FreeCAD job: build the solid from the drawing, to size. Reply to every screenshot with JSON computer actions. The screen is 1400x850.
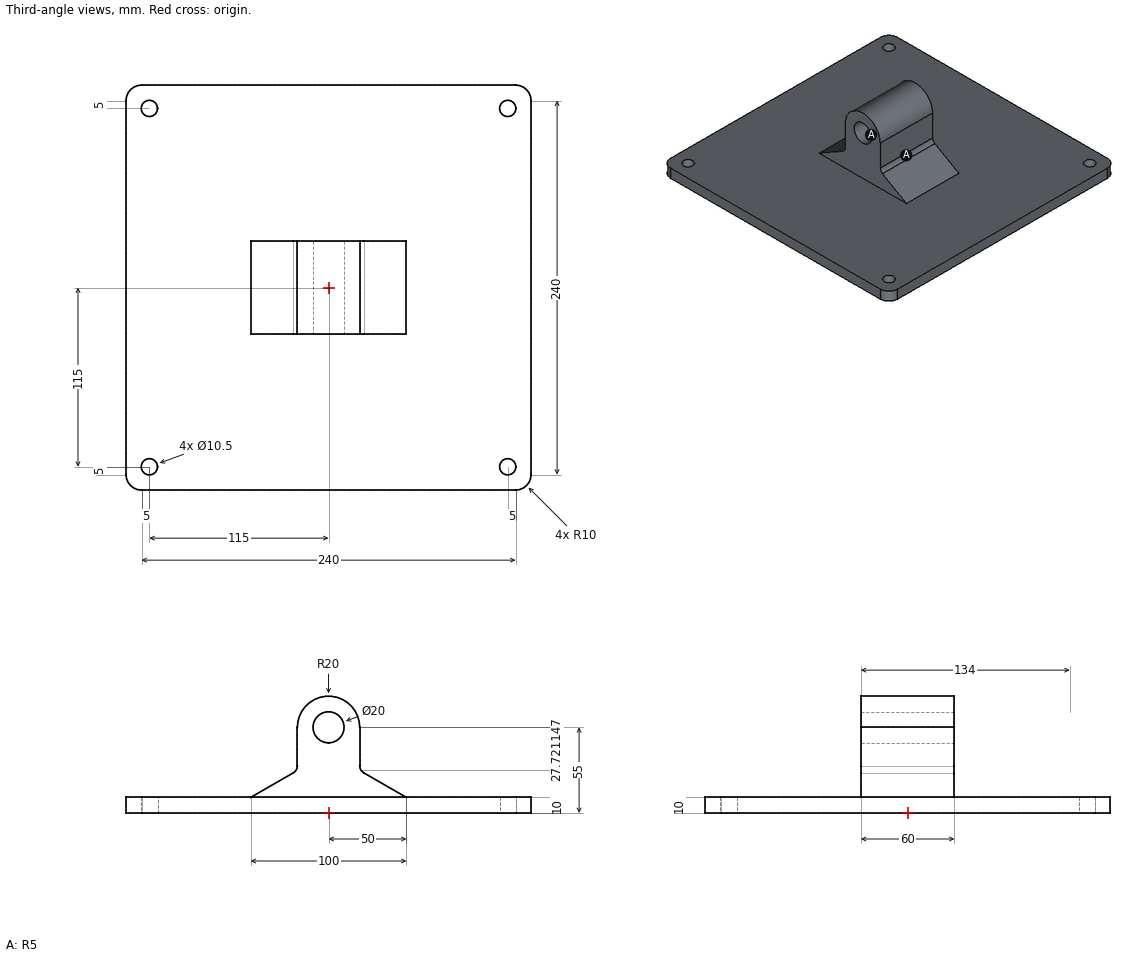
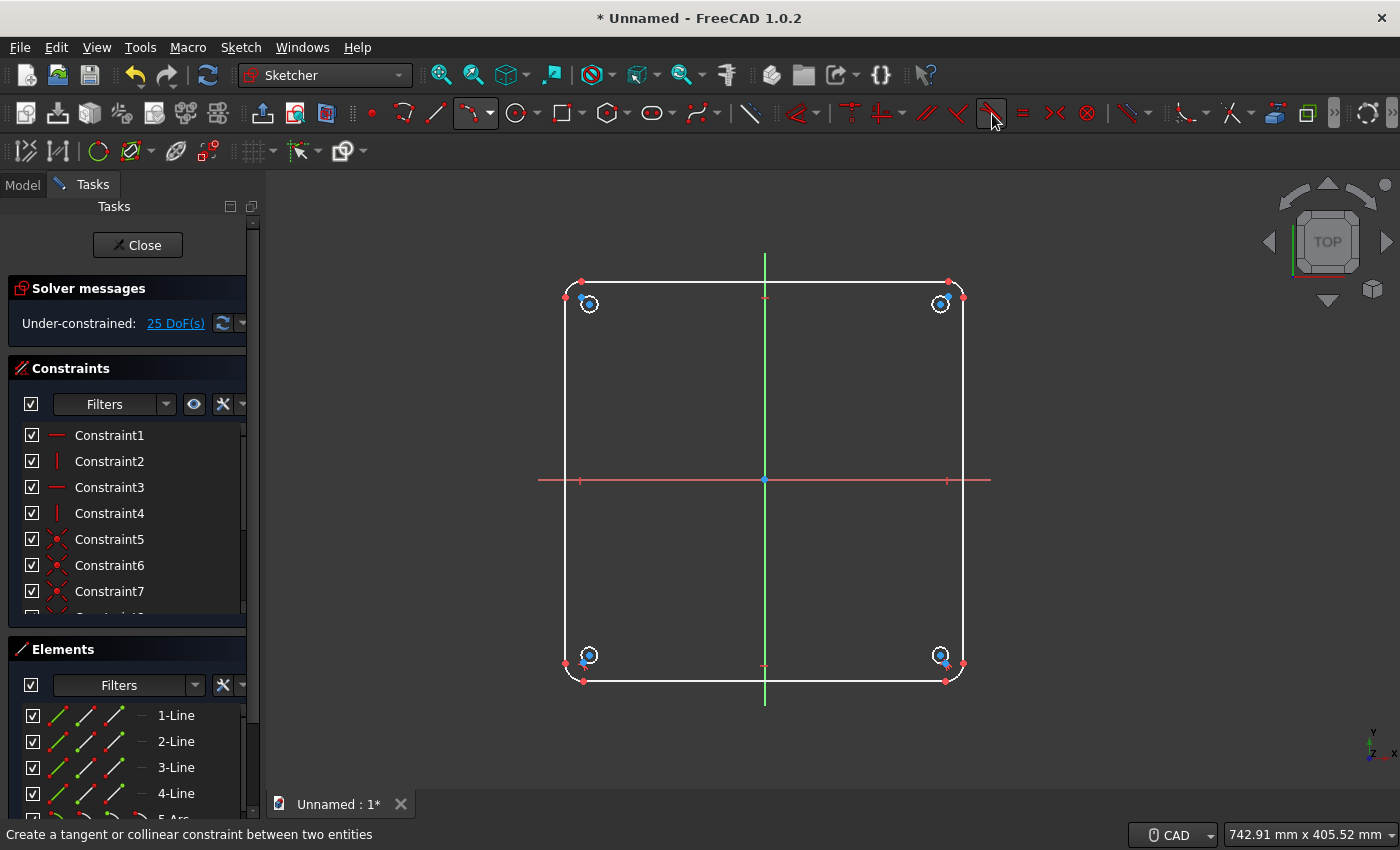
{"action": "left_click", "coordinate": [963, 554]}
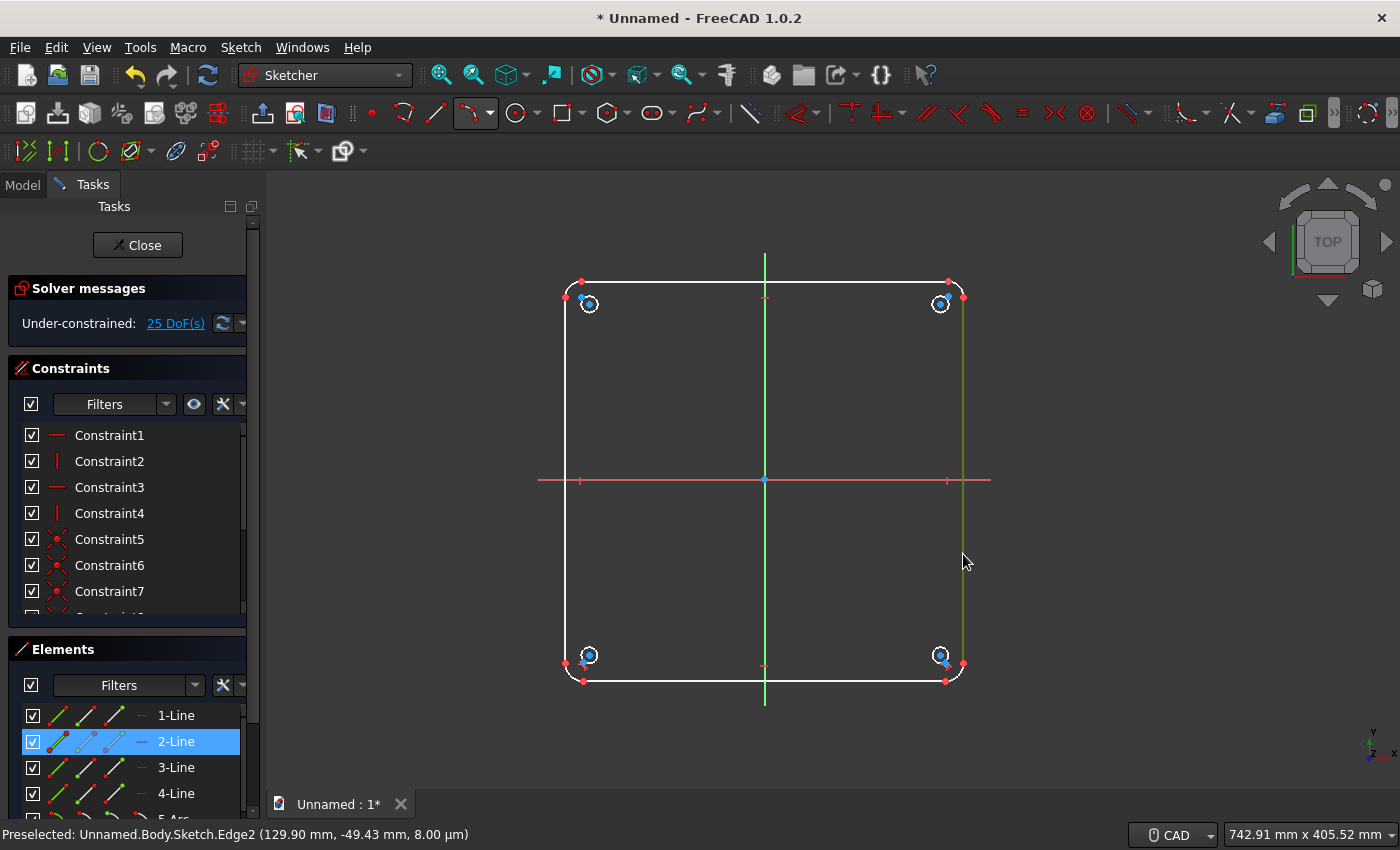
{"action": "left_click", "coordinate": [959, 287]}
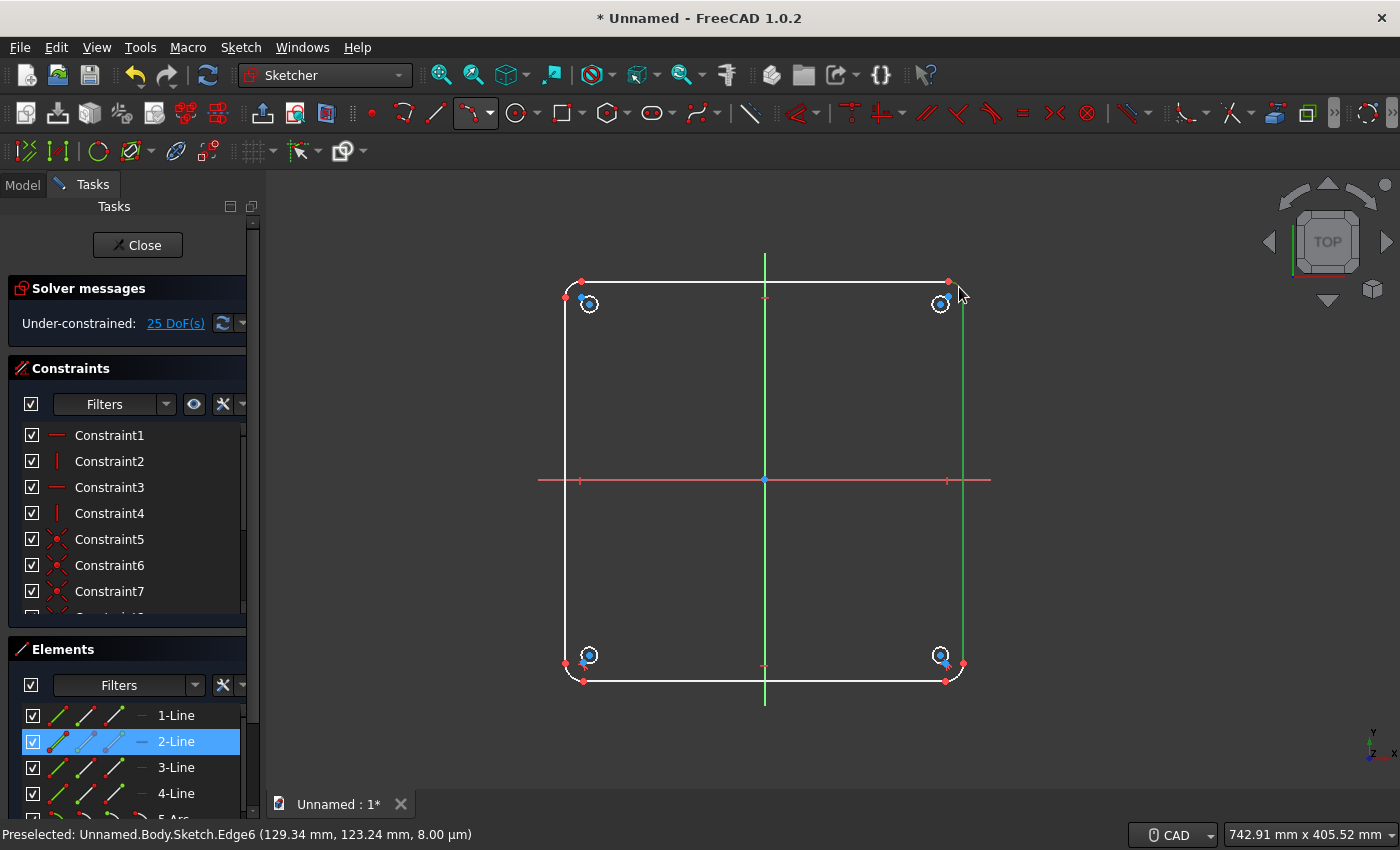
{"action": "left_click", "coordinate": [992, 114]}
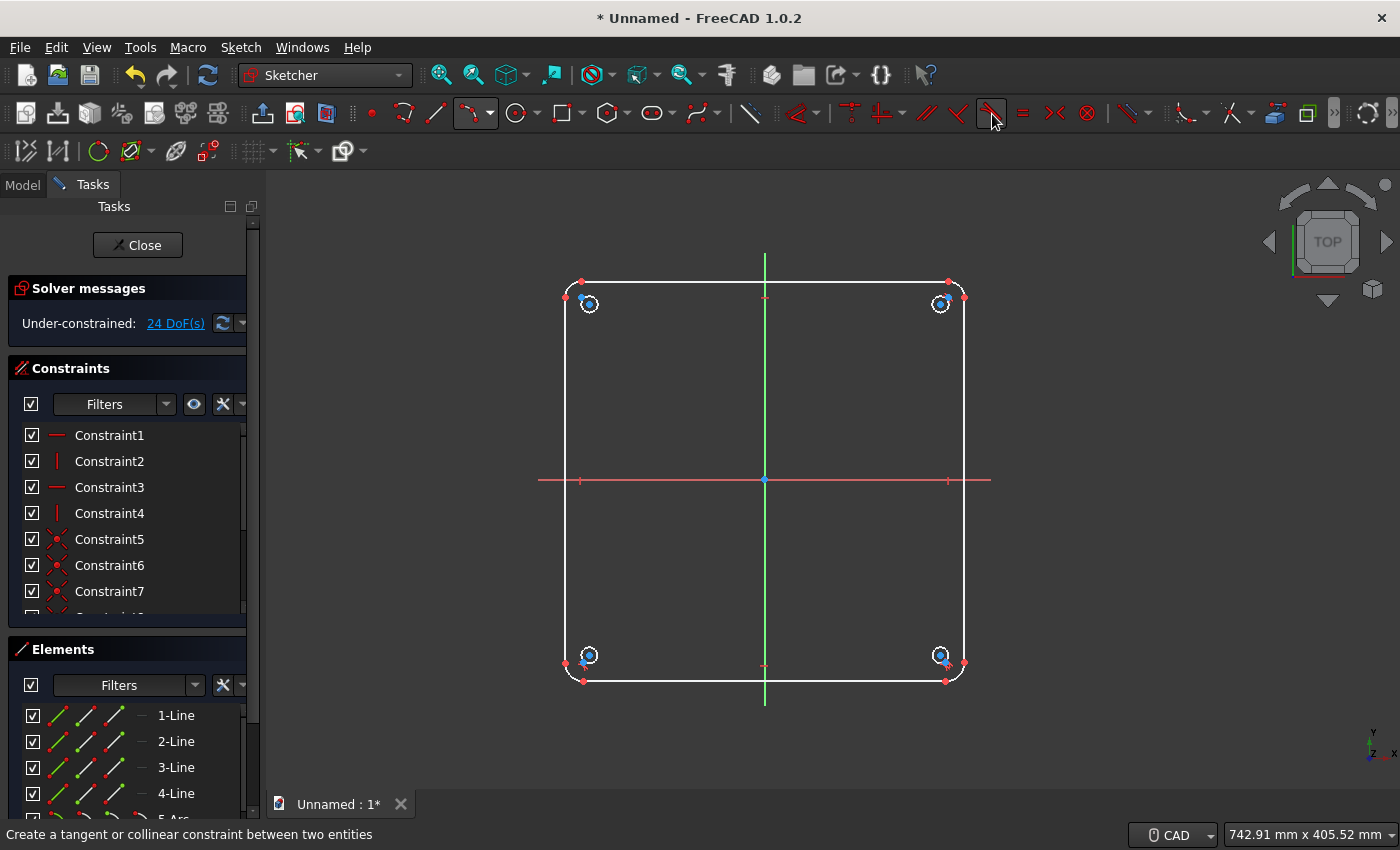
{"action": "left_click", "coordinate": [839, 282]}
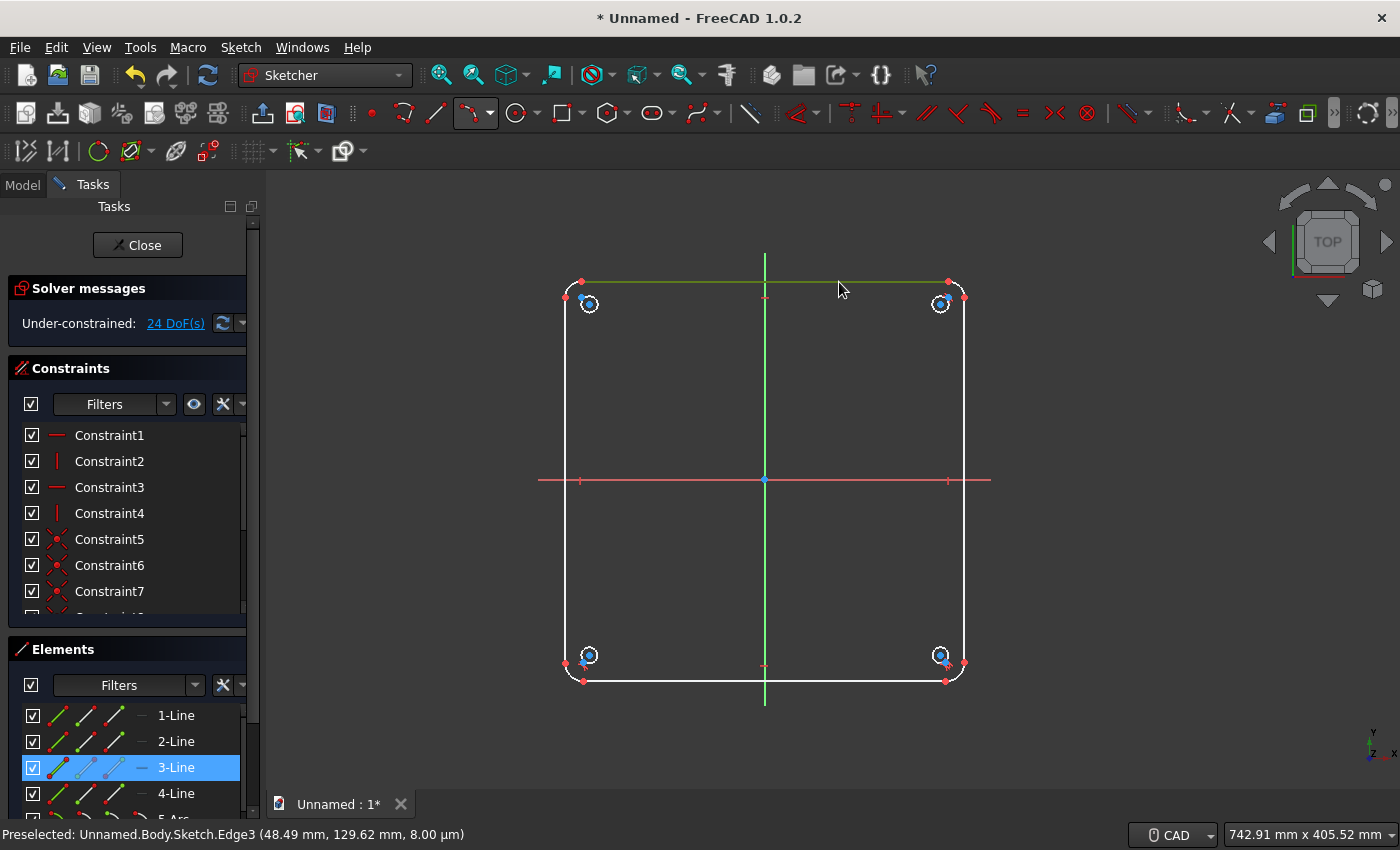
{"action": "left_click", "coordinate": [960, 286]}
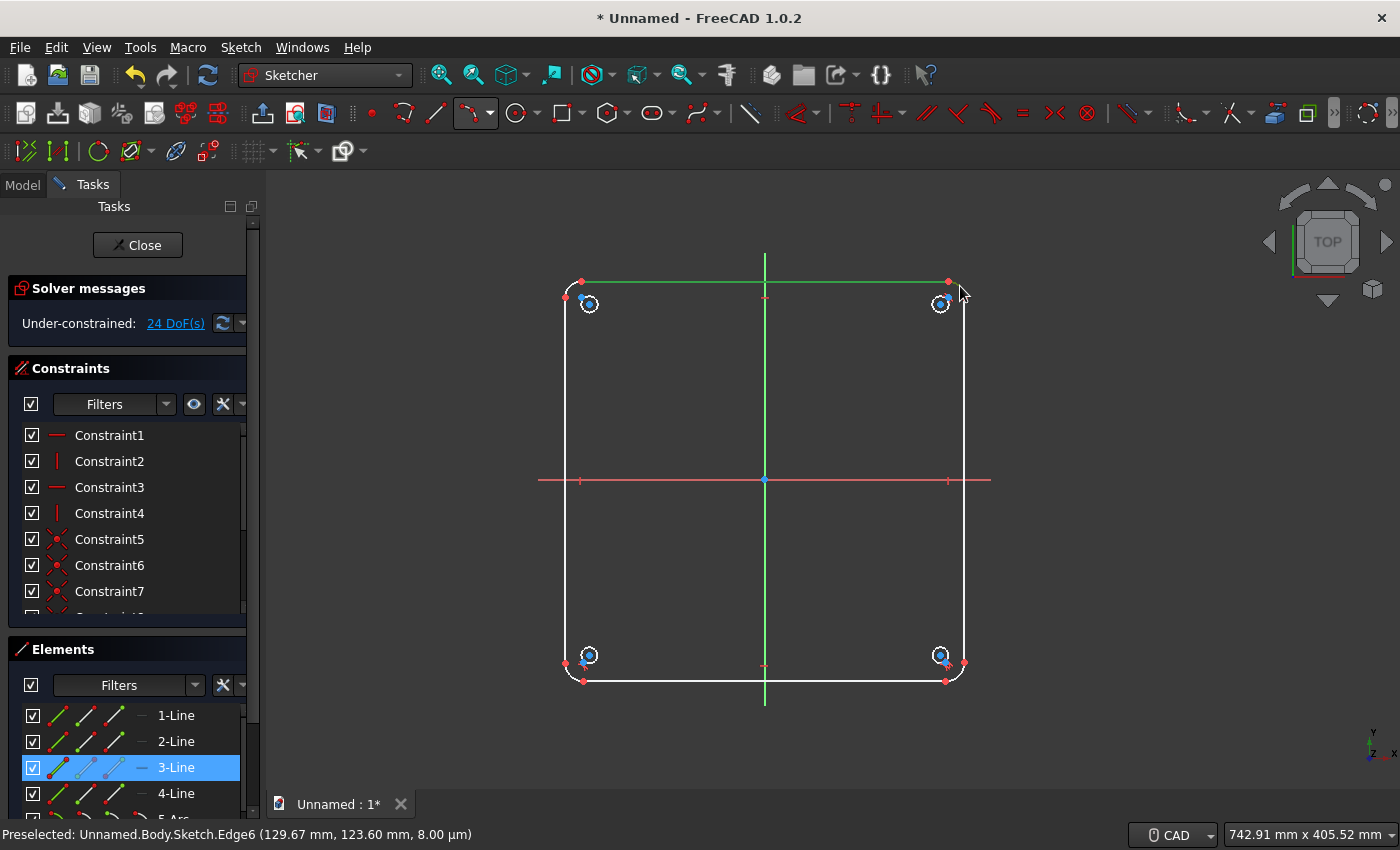
{"action": "left_click", "coordinate": [992, 114]}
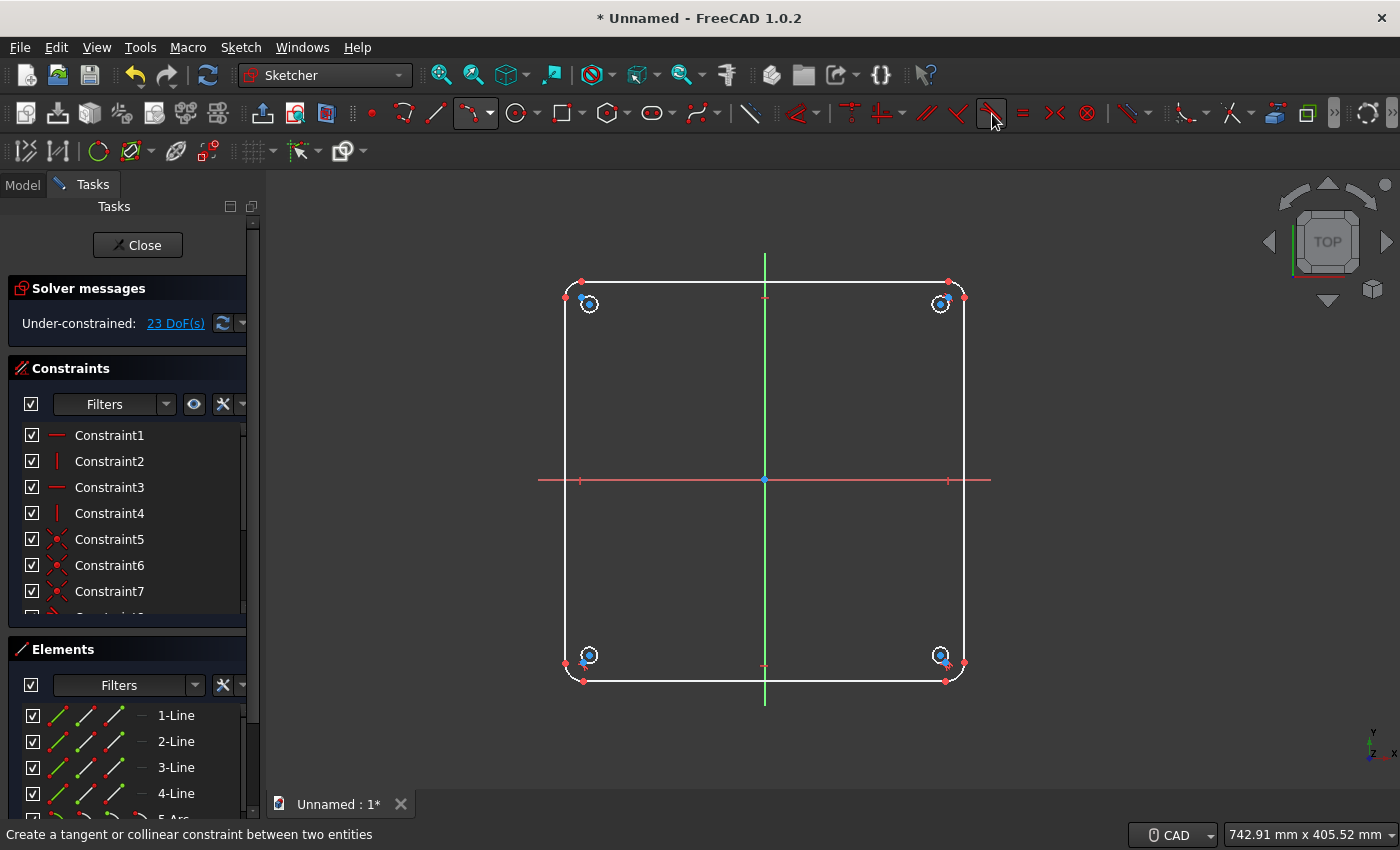
{"action": "left_click", "coordinate": [838, 282]}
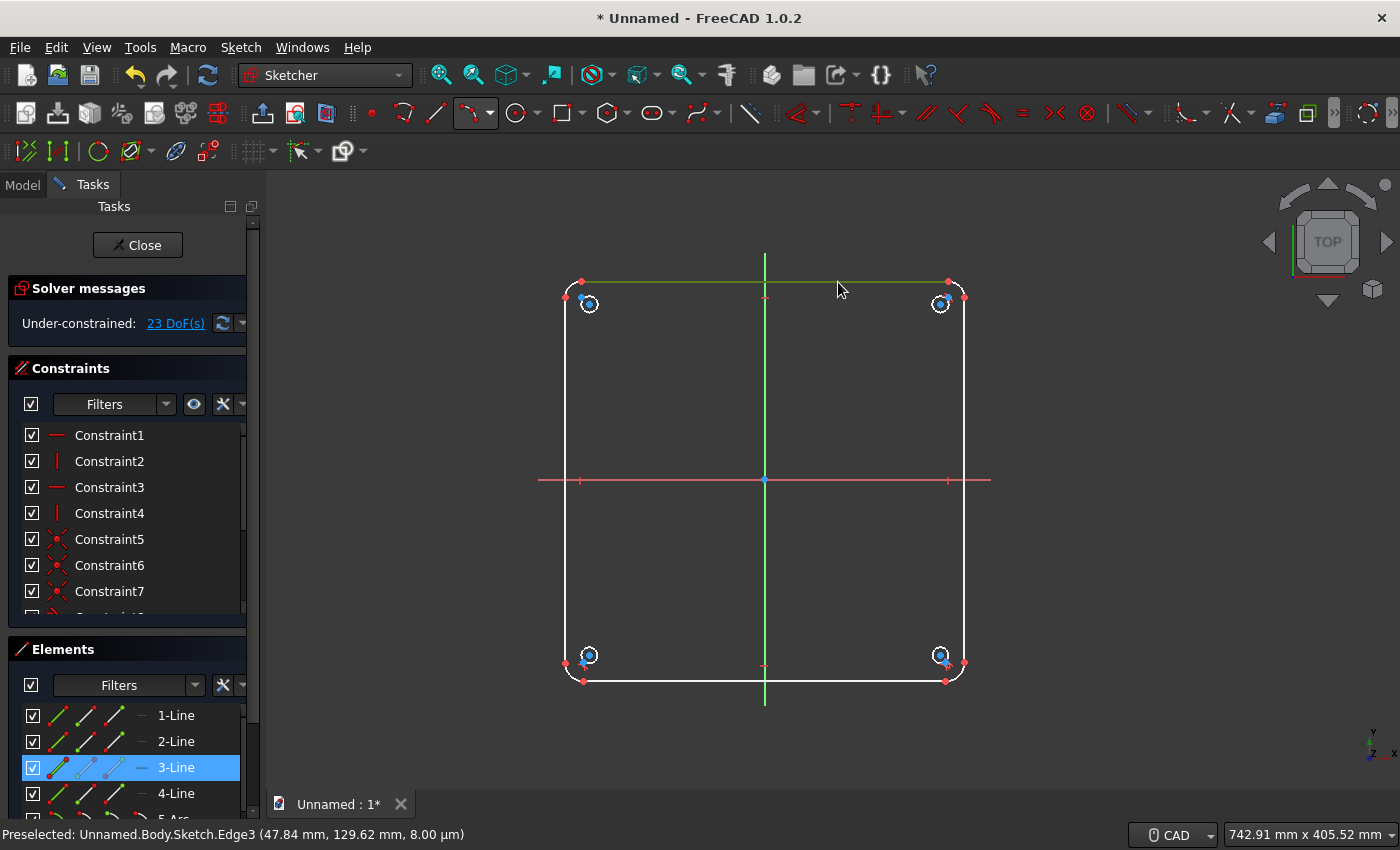
{"action": "left_click", "coordinate": [570, 286]}